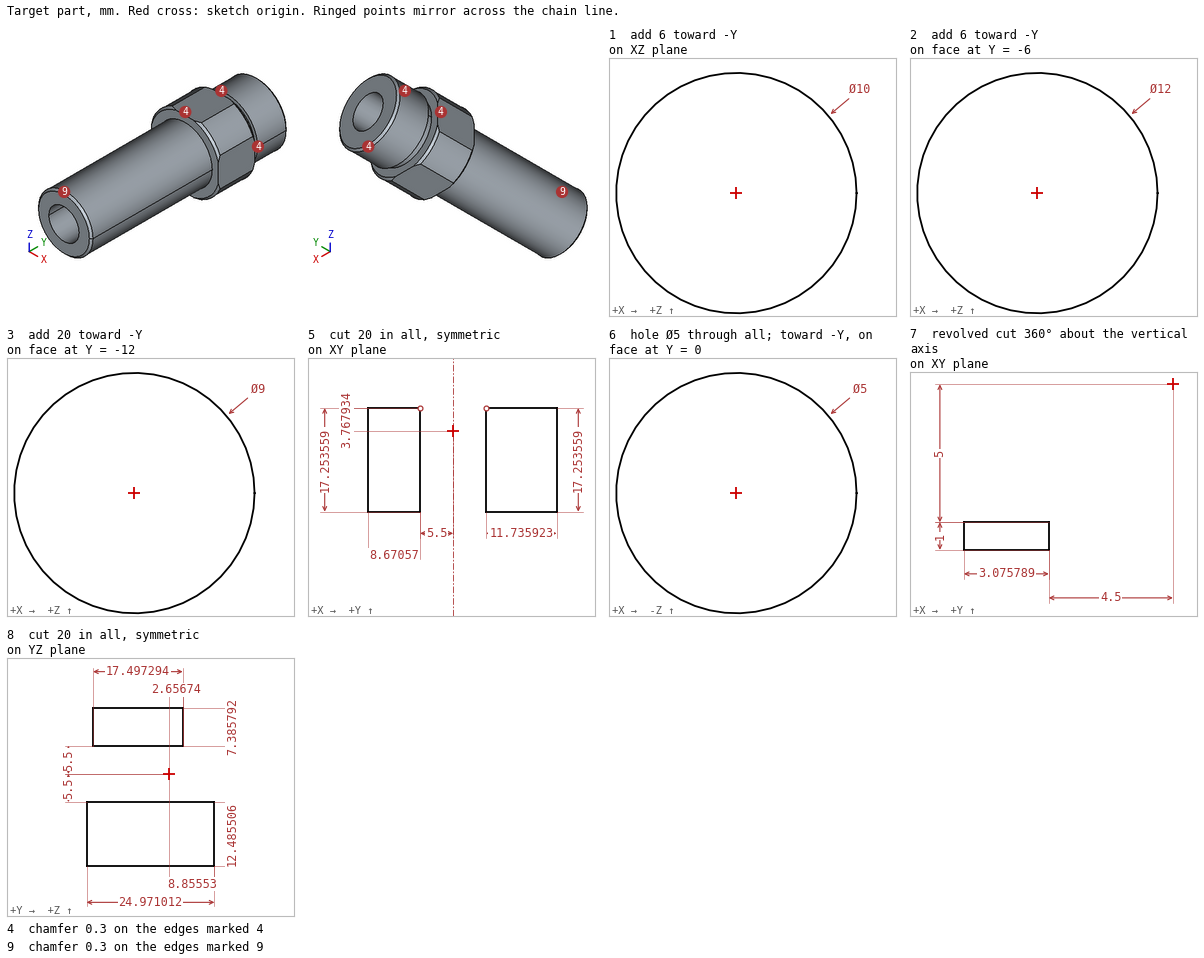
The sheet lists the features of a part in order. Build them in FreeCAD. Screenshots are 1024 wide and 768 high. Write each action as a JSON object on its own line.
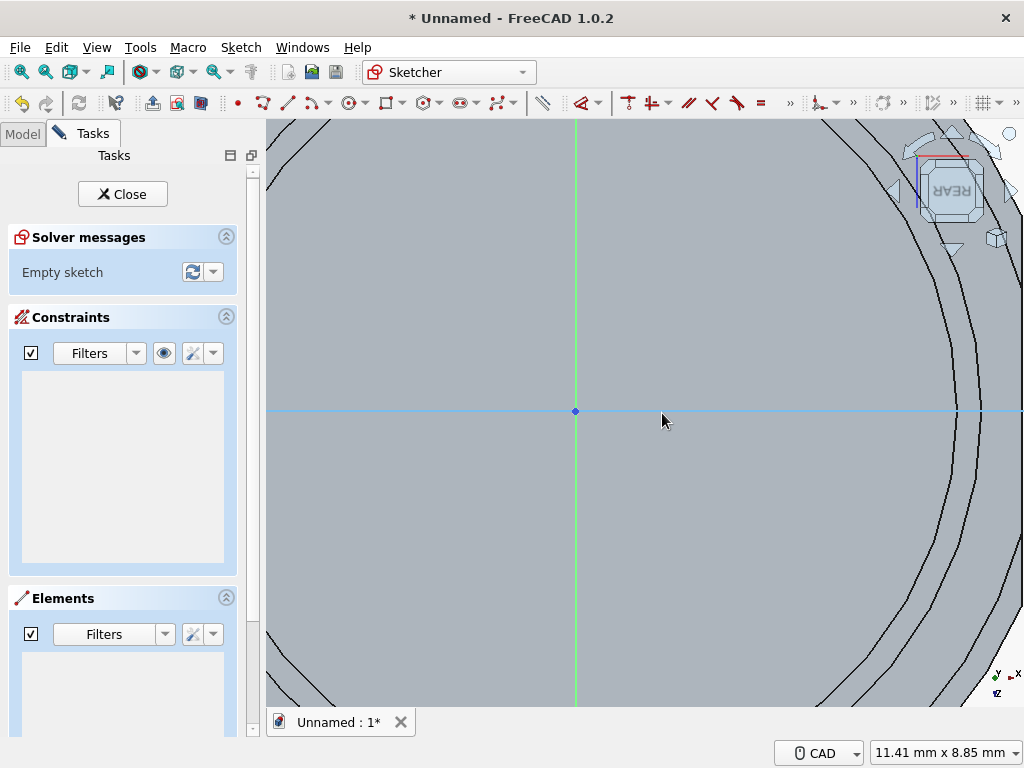
{"action": "key", "text": "g c"}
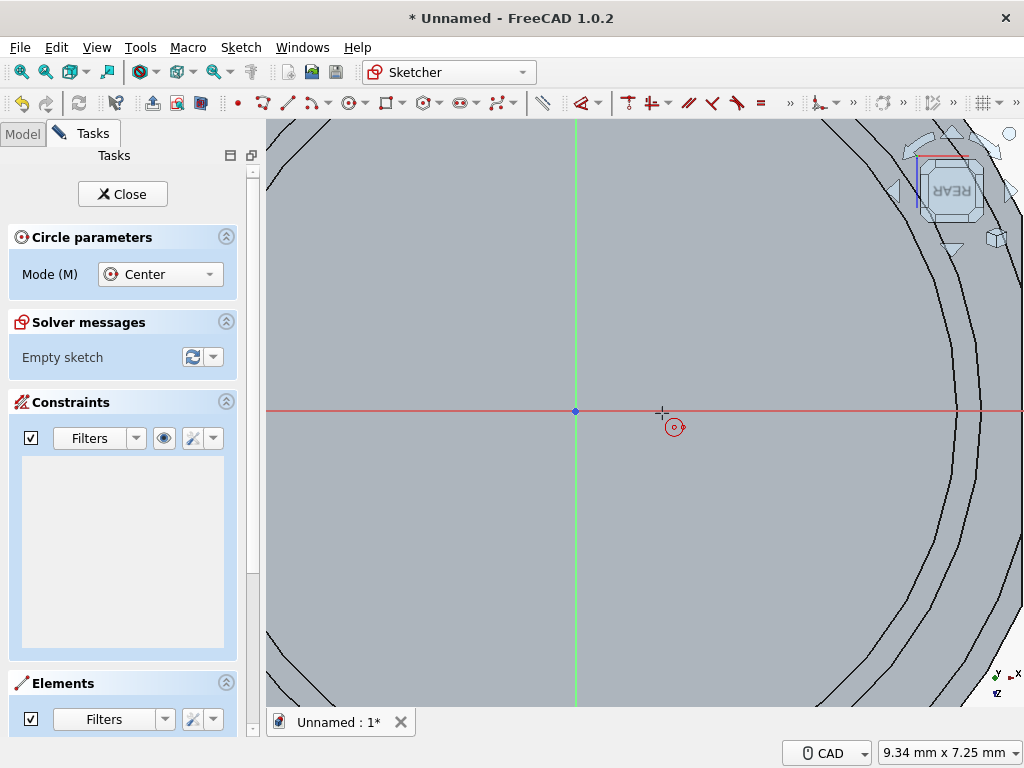
{"action": "left_click", "coordinate": [576, 411]}
{"action": "mouse_move", "coordinate": [719, 268]}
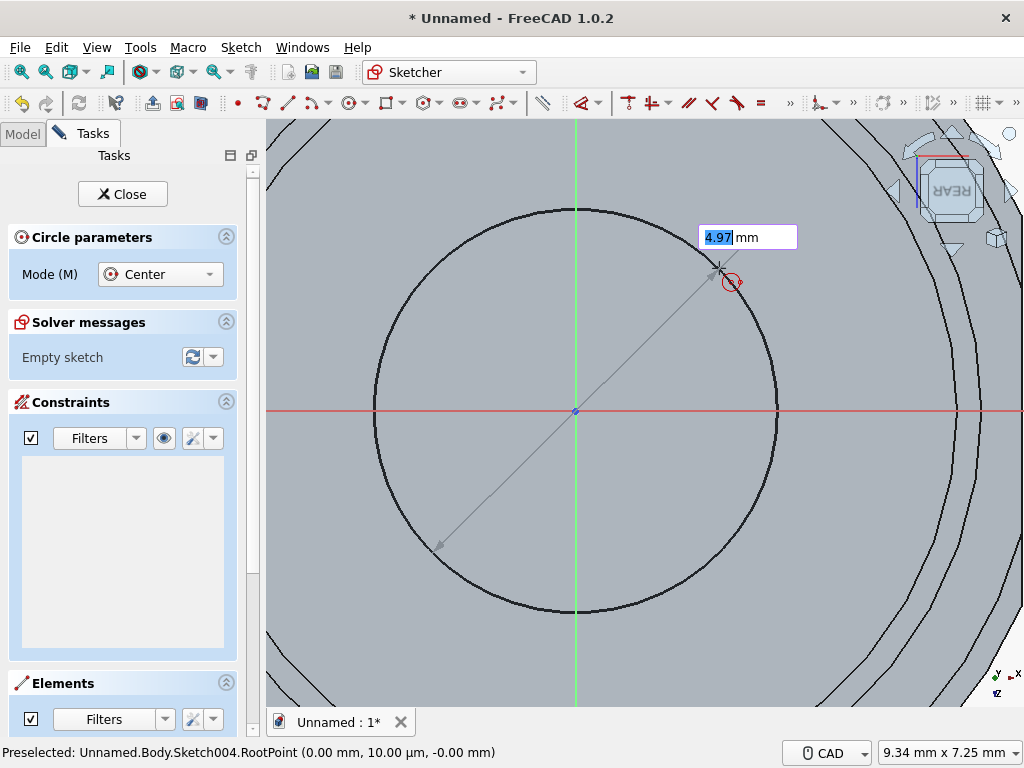
{"action": "type", "text": "5"}
{"action": "key", "text": "Return"}
{"action": "key", "text": "Escape"}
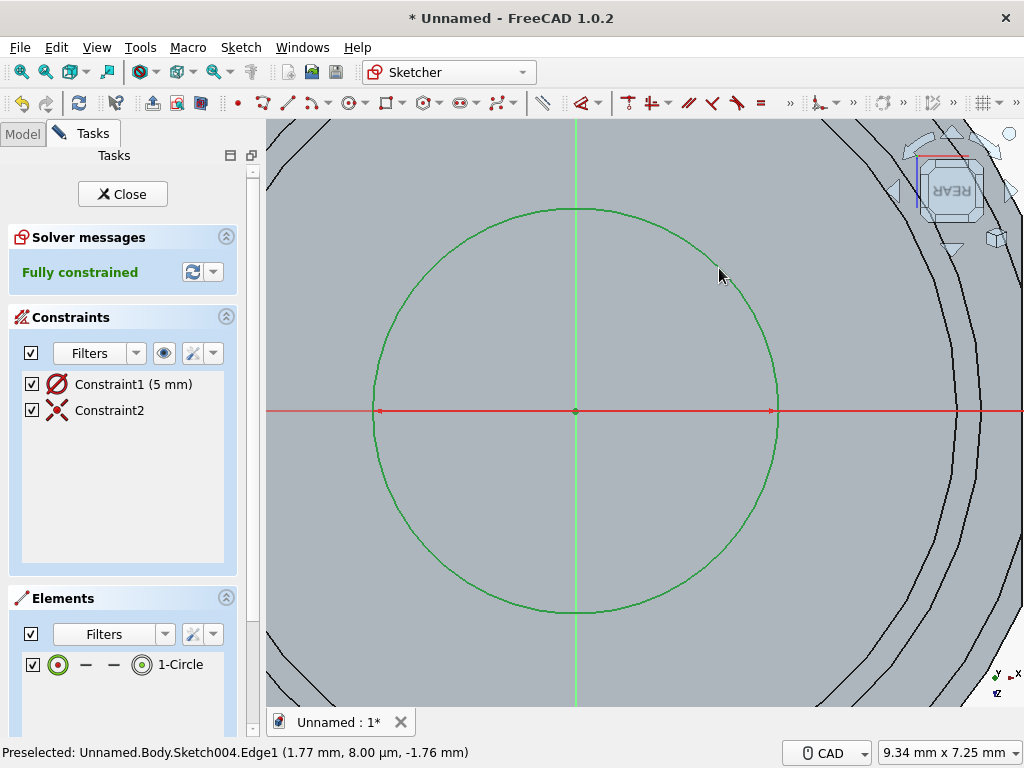
{"action": "left_click", "coordinate": [123, 194]}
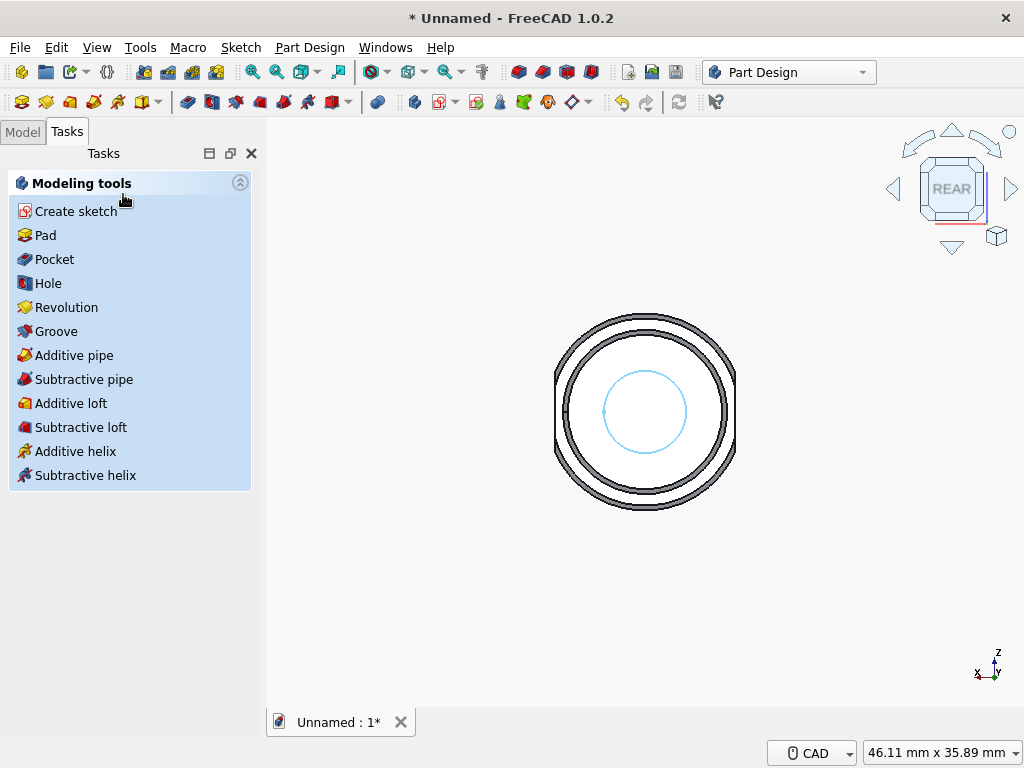
{"action": "left_click", "coordinate": [212, 102]}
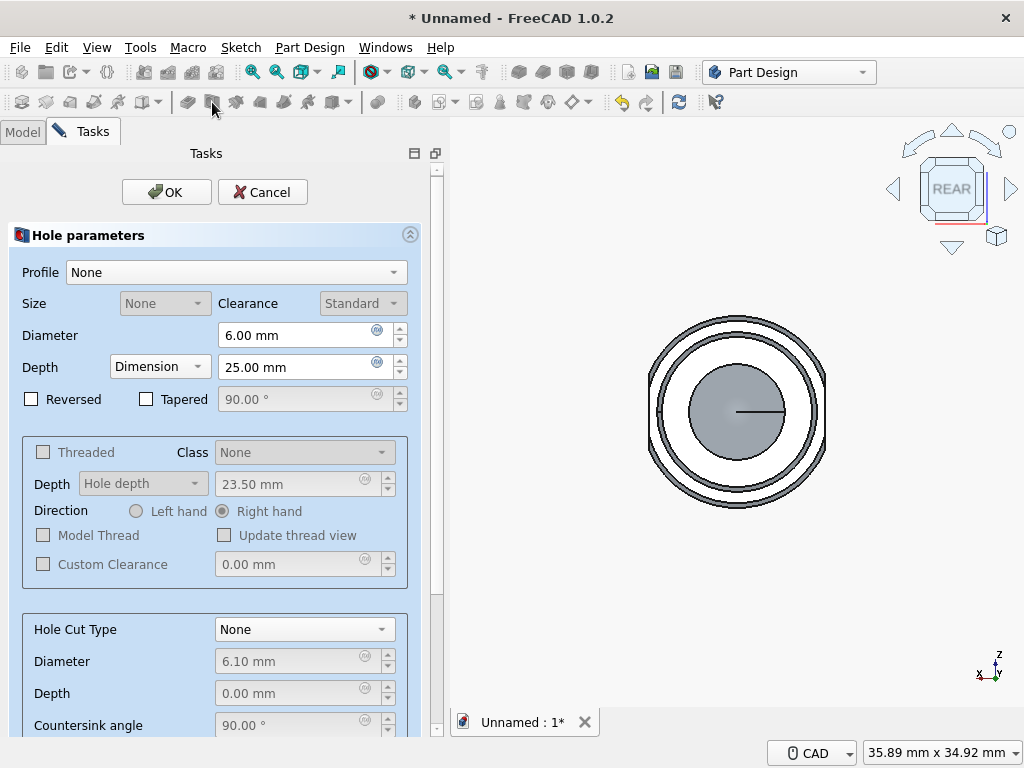
{"action": "triple_click", "coordinate": [305, 335]}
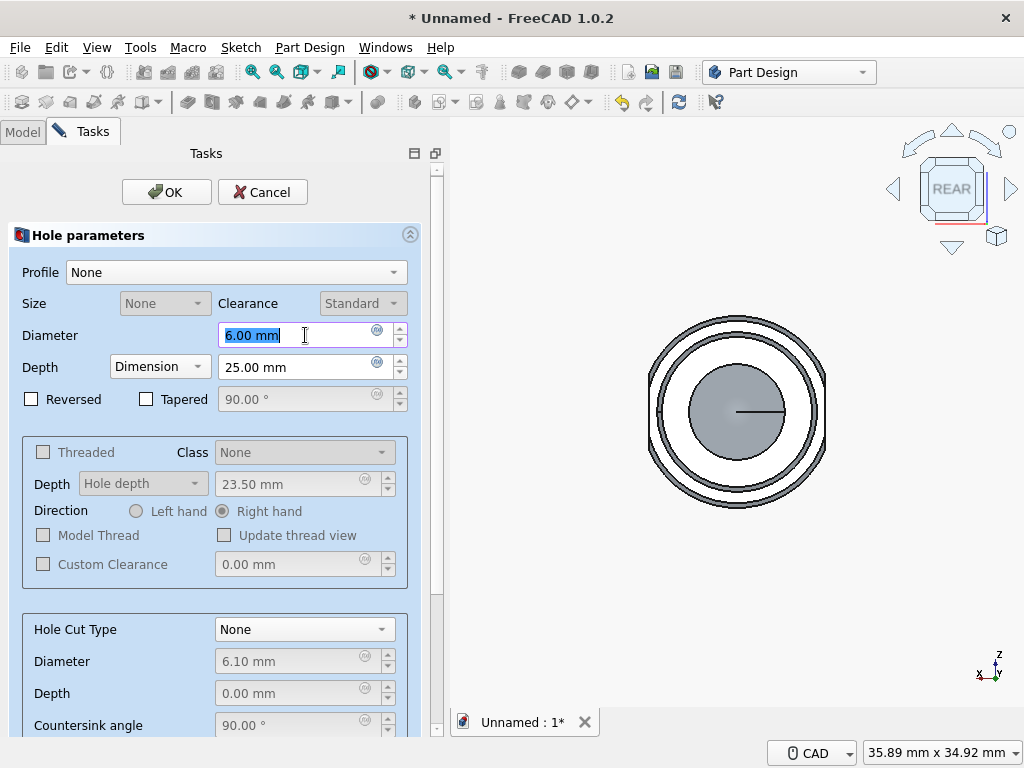
{"action": "type", "text": "5"}
{"action": "key", "text": "Tab"}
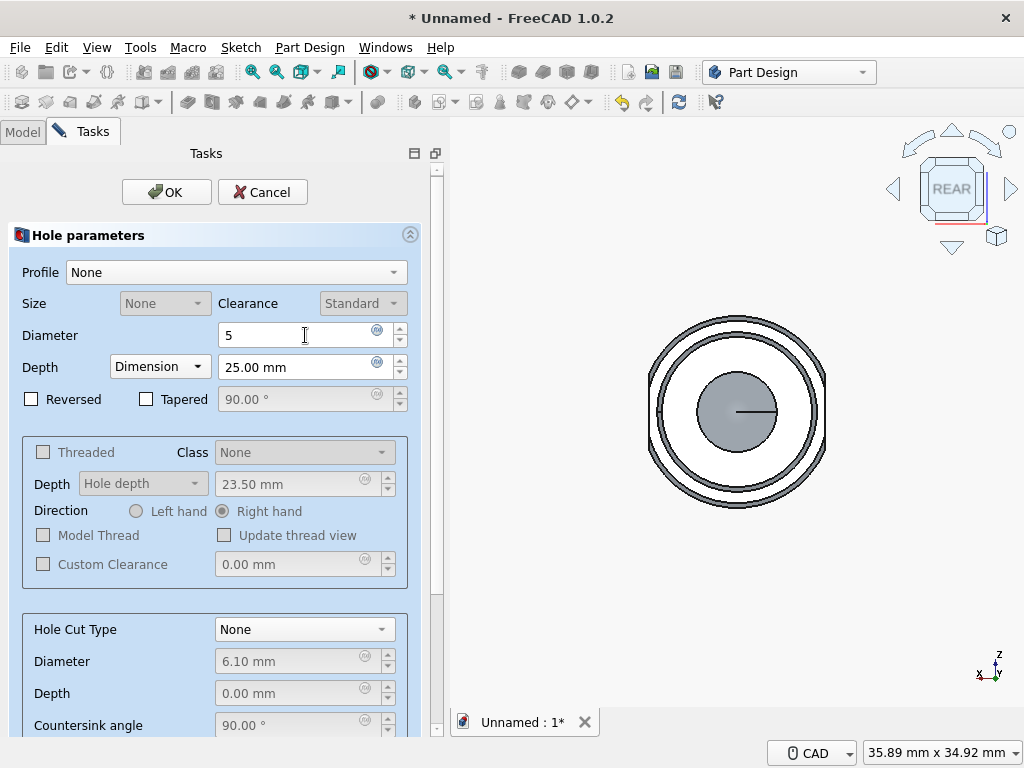
{"action": "left_click", "coordinate": [161, 366]}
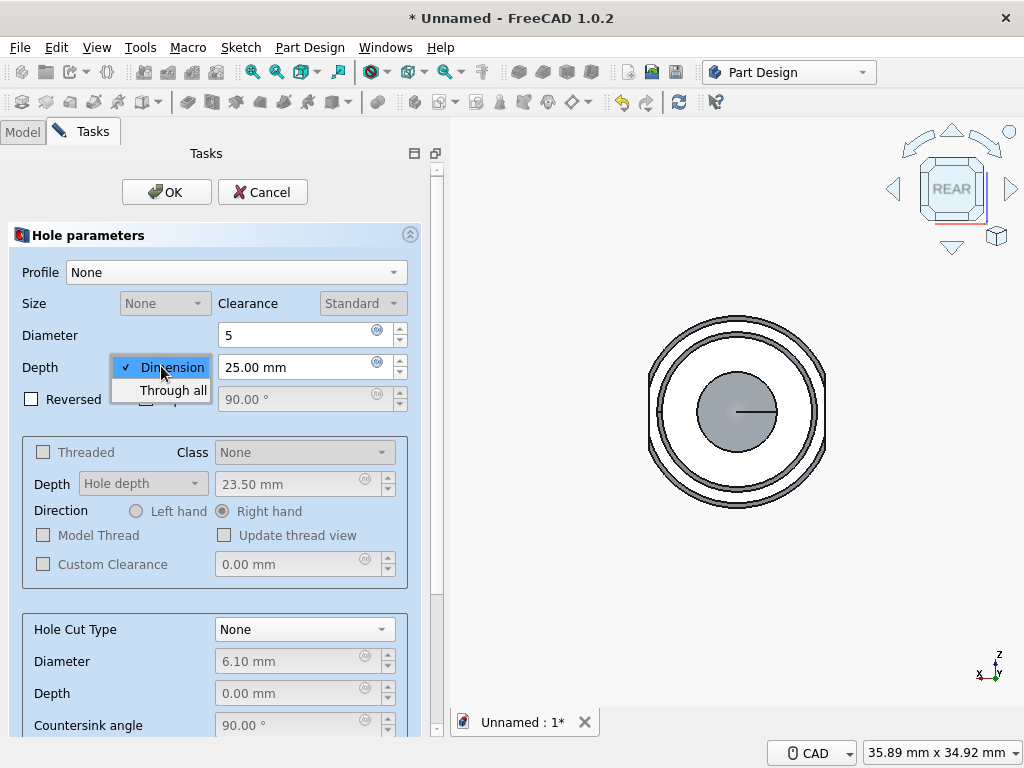
{"action": "left_click", "coordinate": [160, 390]}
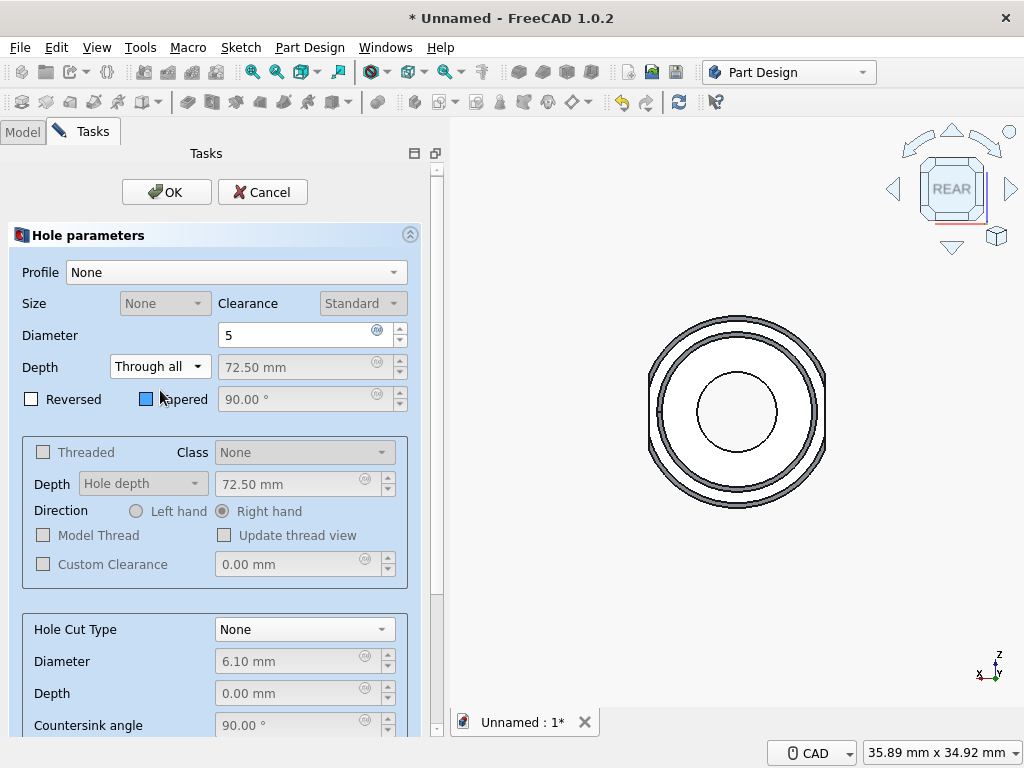
{"action": "left_click", "coordinate": [167, 192]}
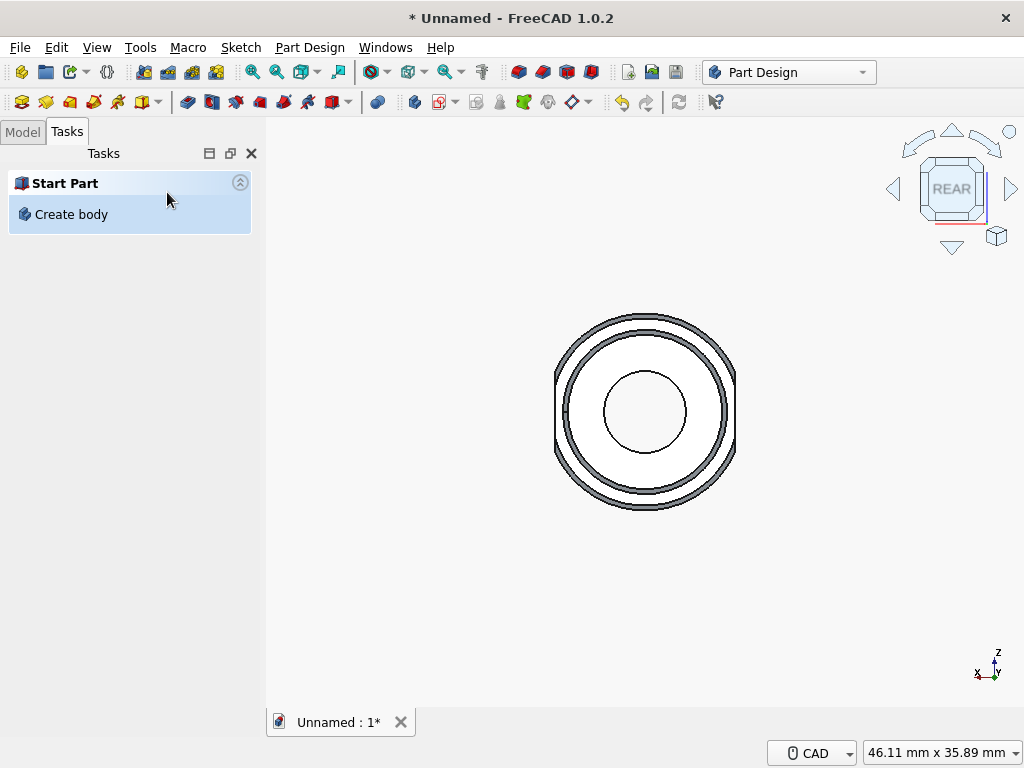
{"action": "key", "text": "v f"}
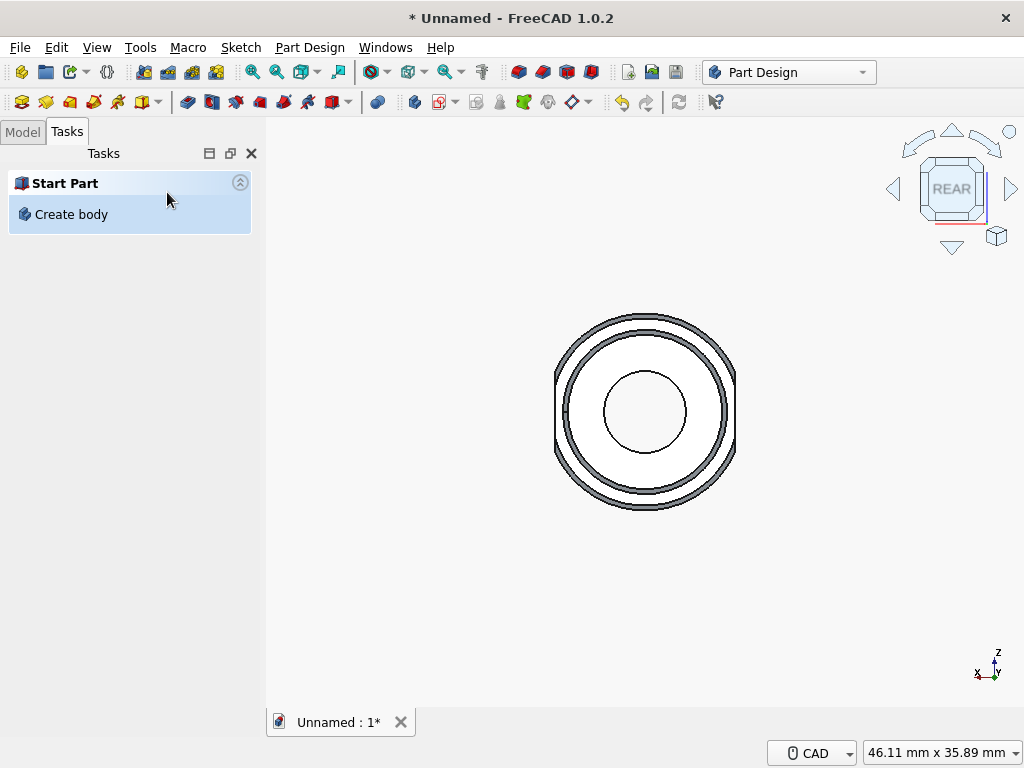
{"action": "left_click", "coordinate": [440, 102]}